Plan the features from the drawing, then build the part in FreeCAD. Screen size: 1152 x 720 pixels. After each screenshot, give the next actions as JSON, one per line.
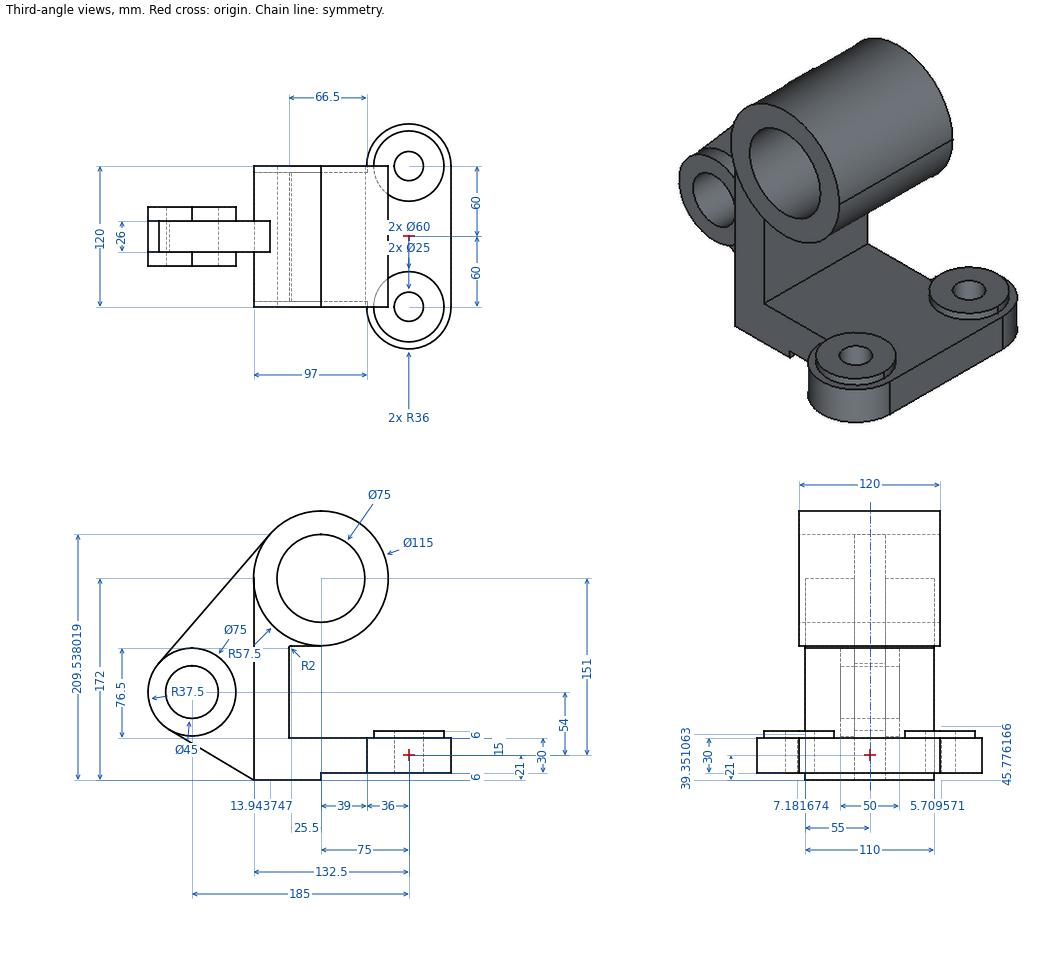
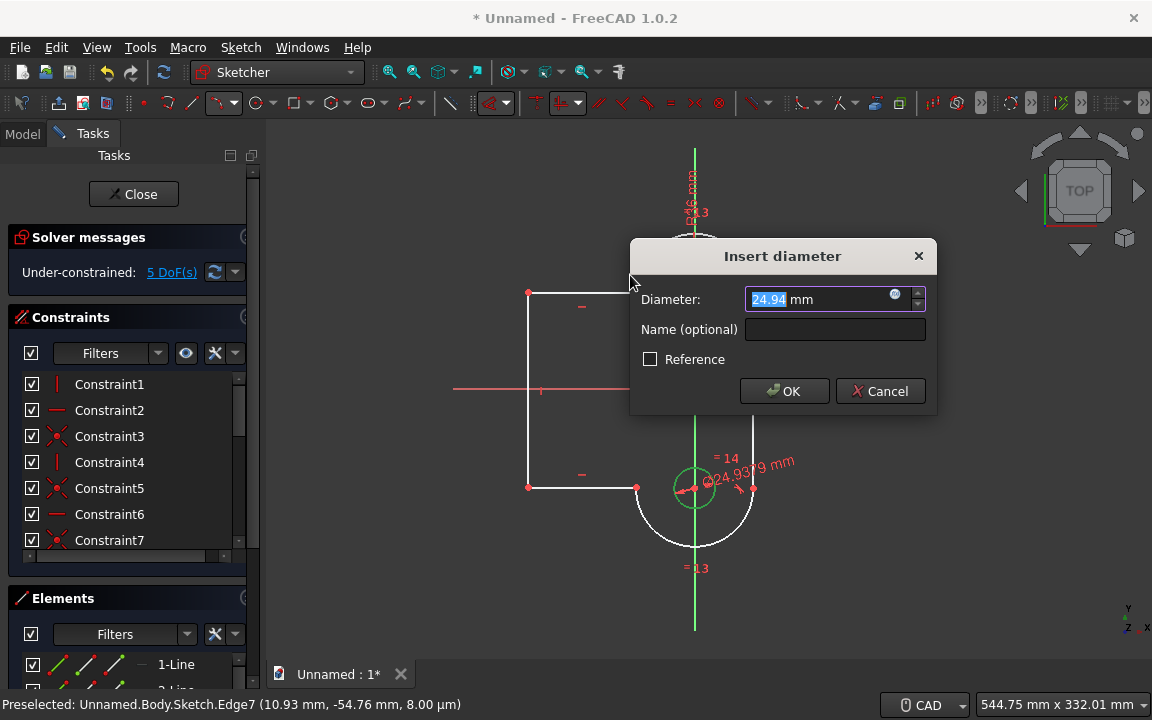
{"action": "type", "text": "25"}
{"action": "key", "text": "Return"}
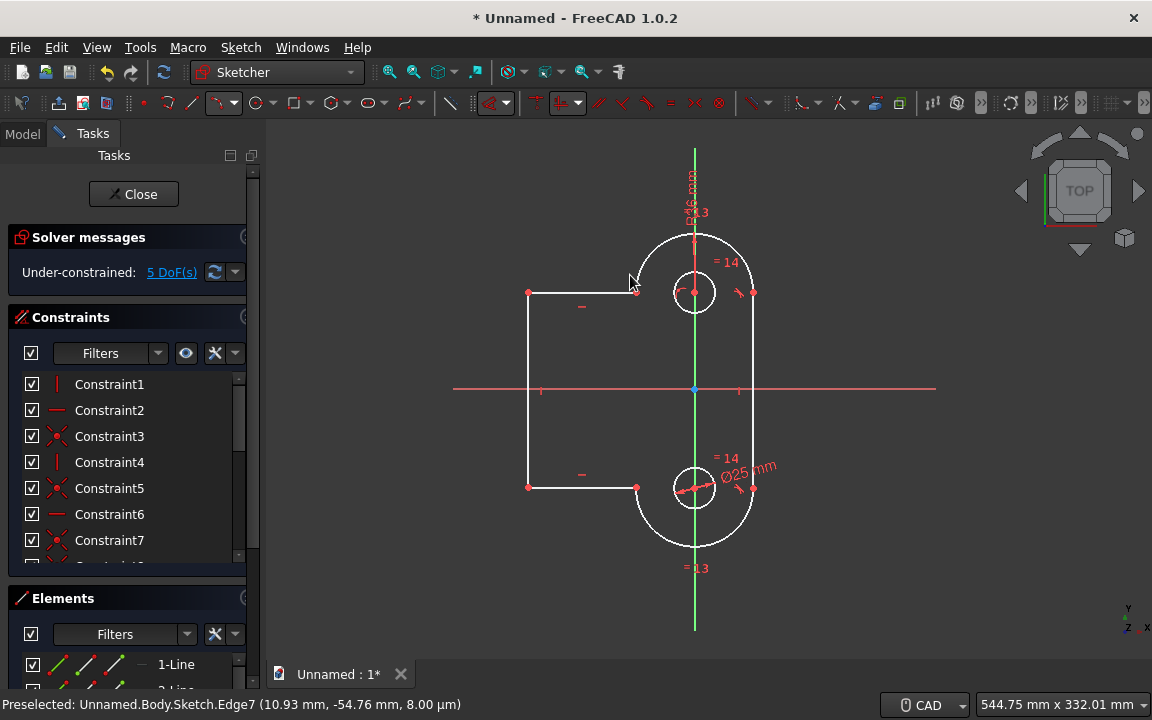
{"action": "left_click", "coordinate": [695, 488]}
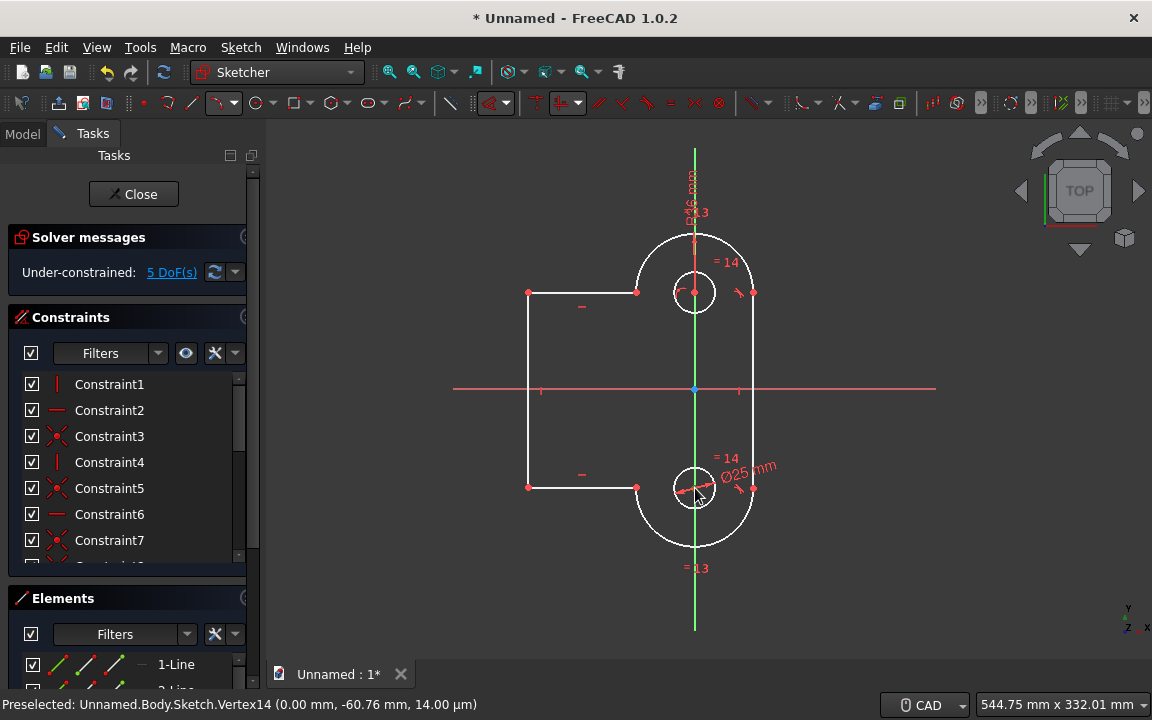
{"action": "key", "text": "i"}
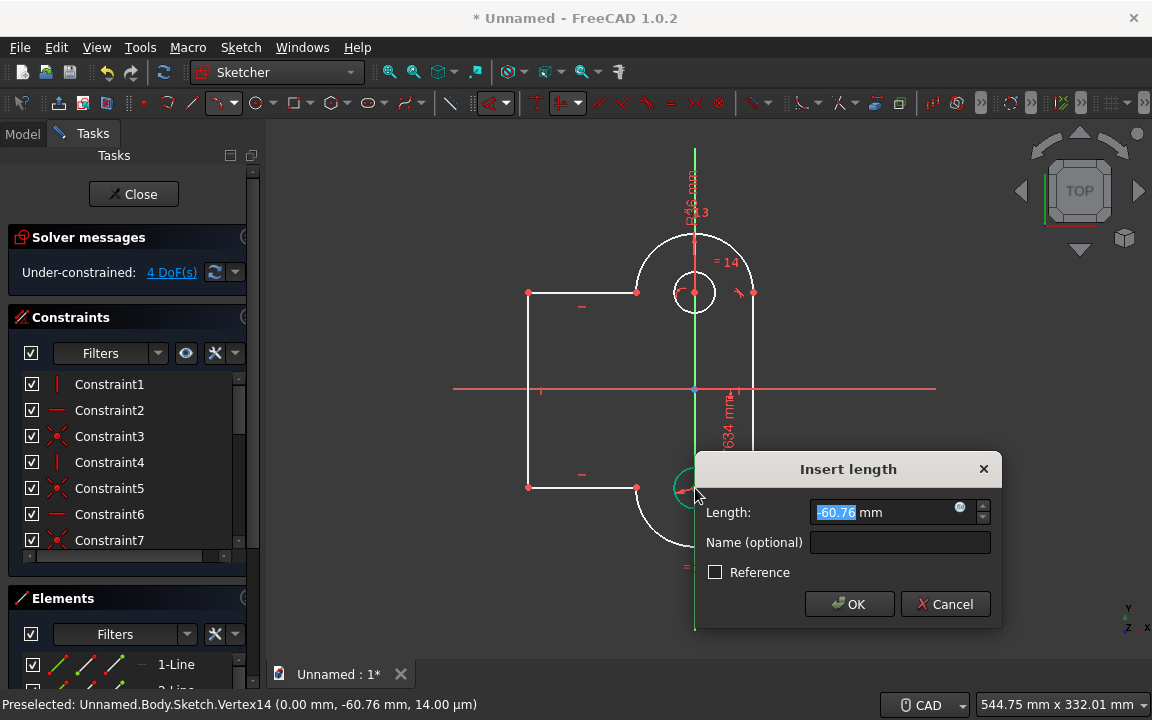
{"action": "type", "text": "-60"}
{"action": "key", "text": "Return"}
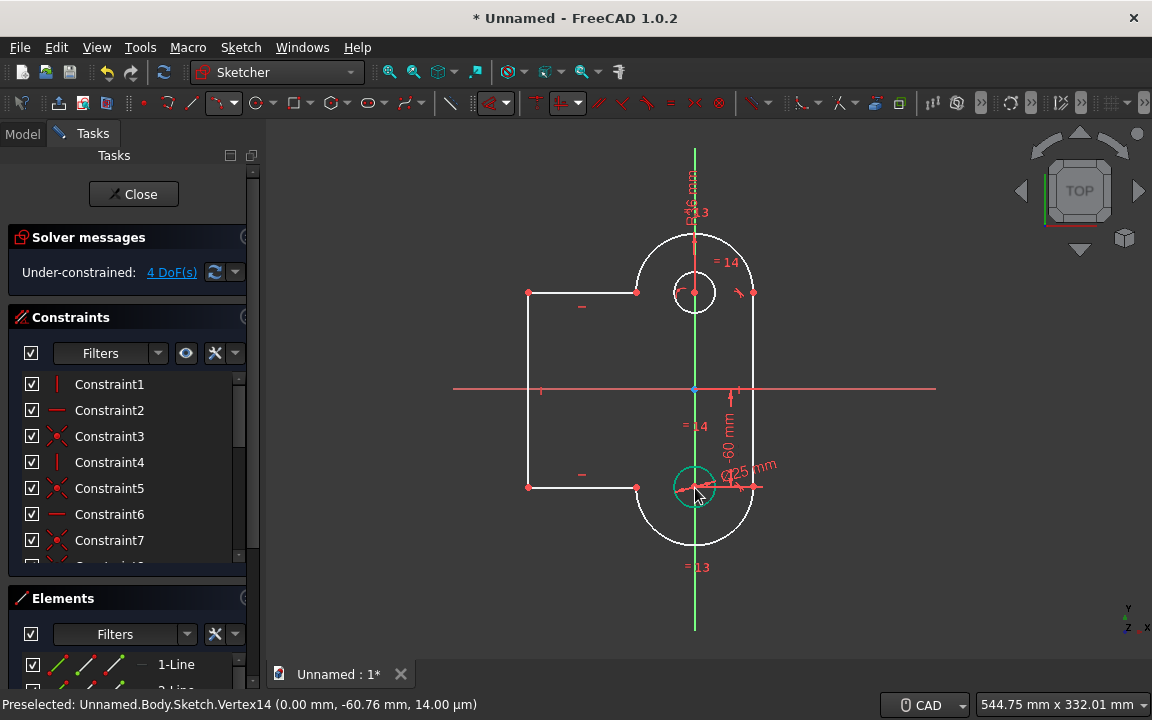
{"action": "left_click", "coordinate": [695, 293]}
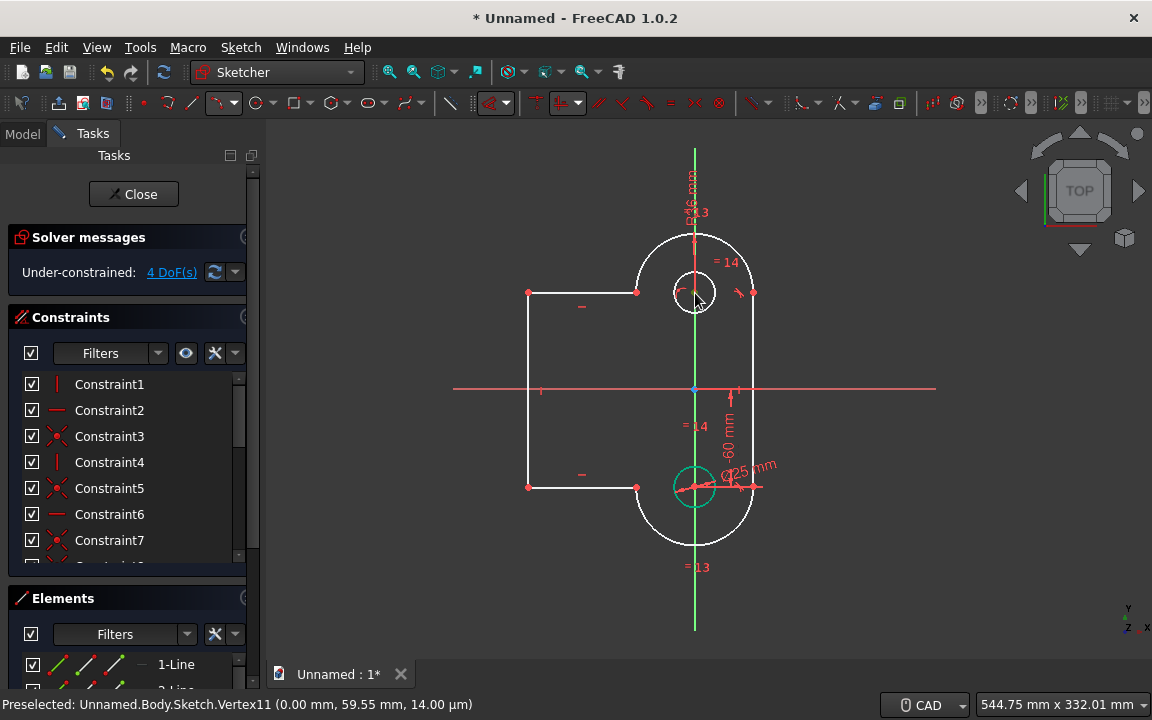
{"action": "key", "text": "i"}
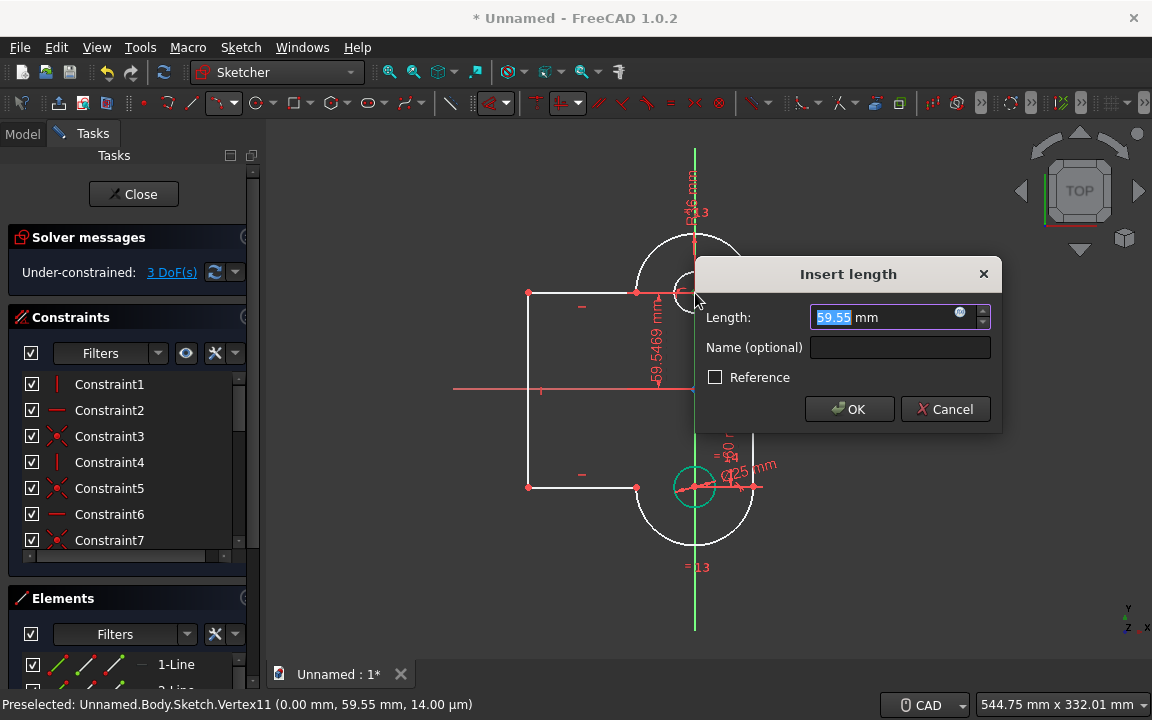
{"action": "type", "text": "60"}
{"action": "key", "text": "Return"}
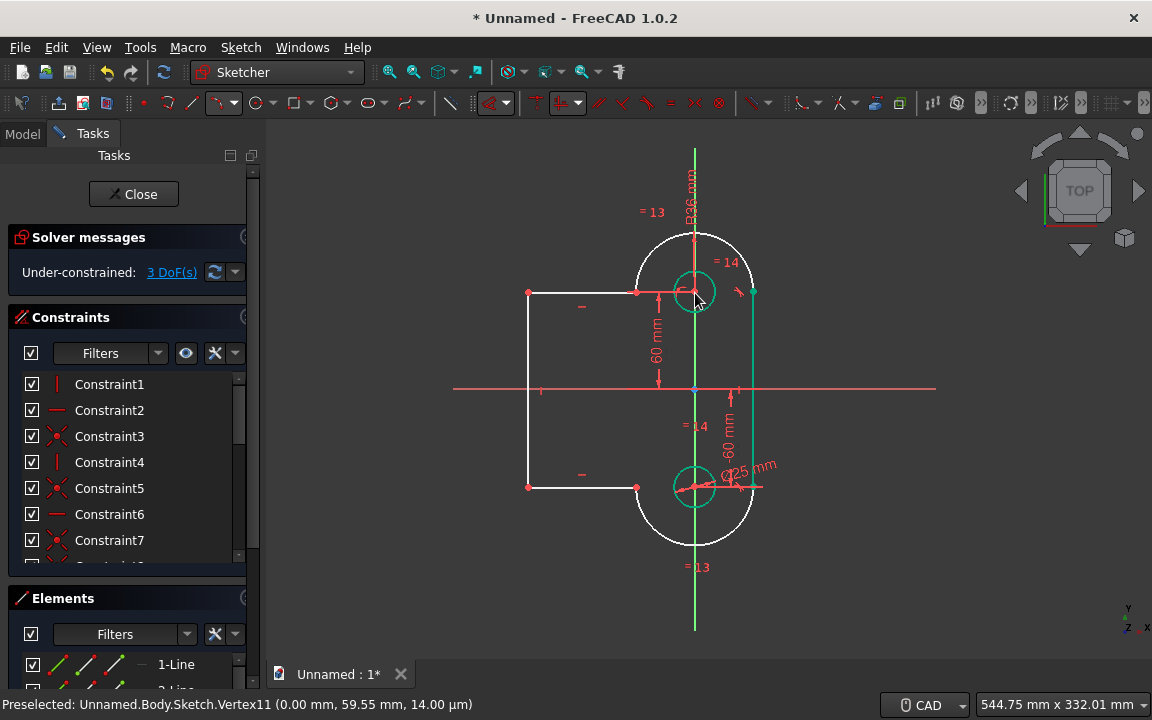
{"action": "left_click", "coordinate": [528, 351]}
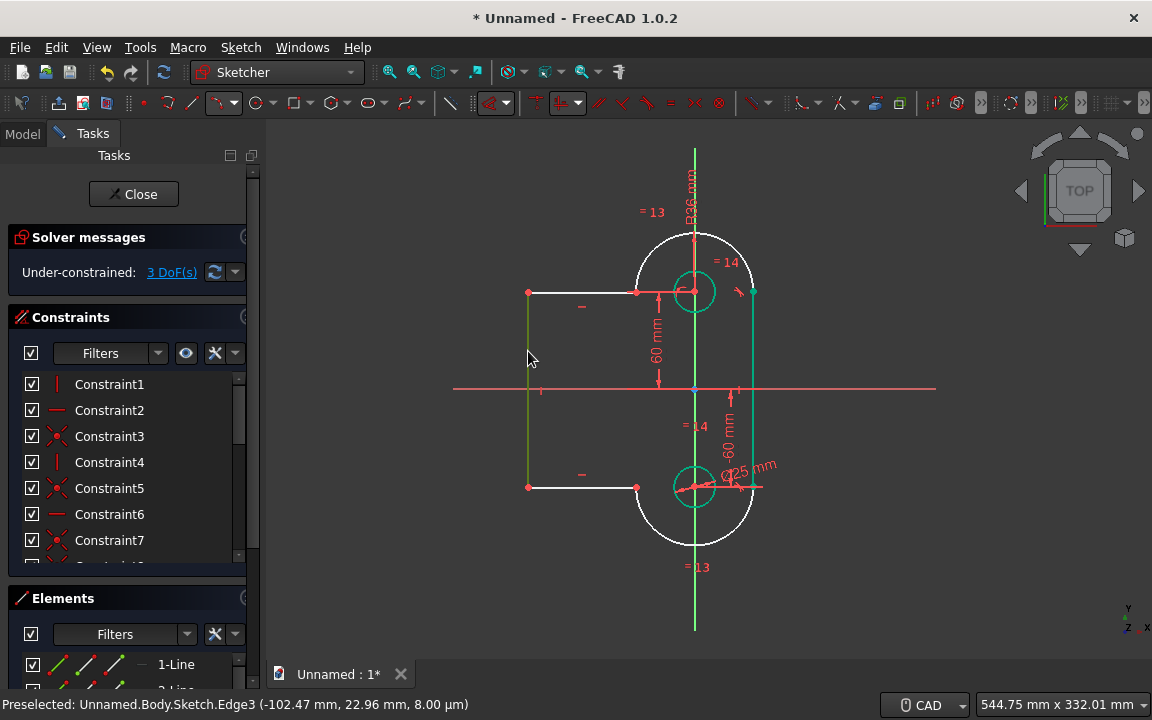
{"action": "key", "text": "i"}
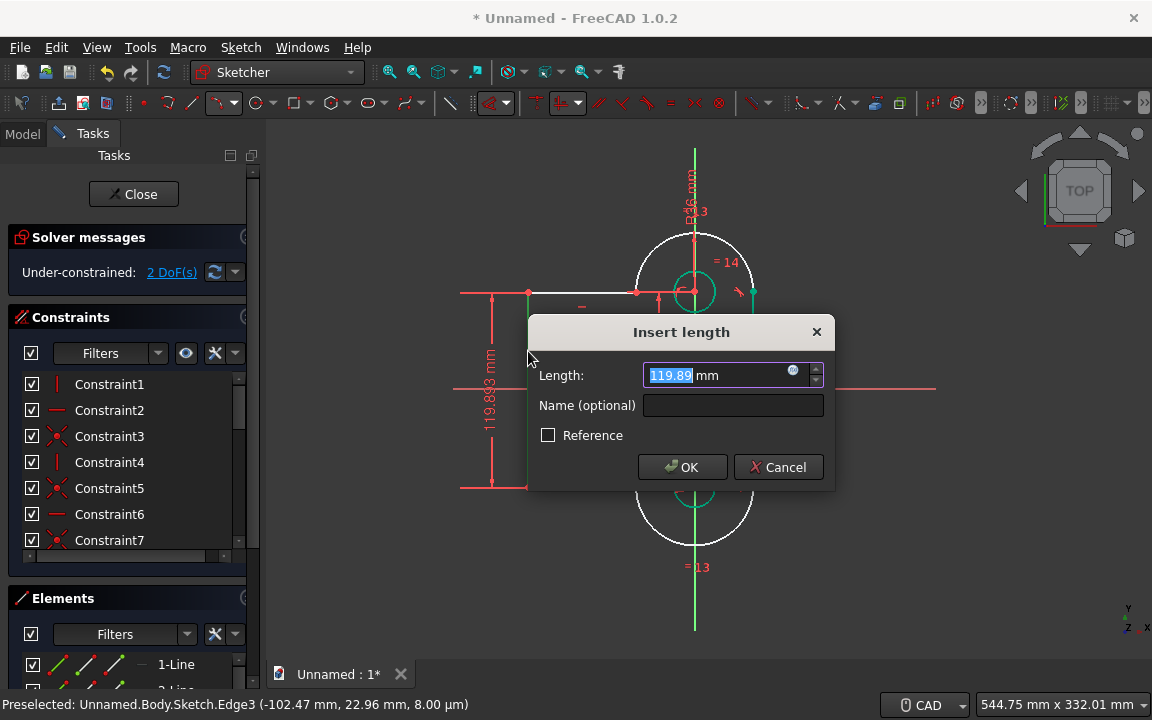
{"action": "type", "text": "120"}
{"action": "key", "text": "Return"}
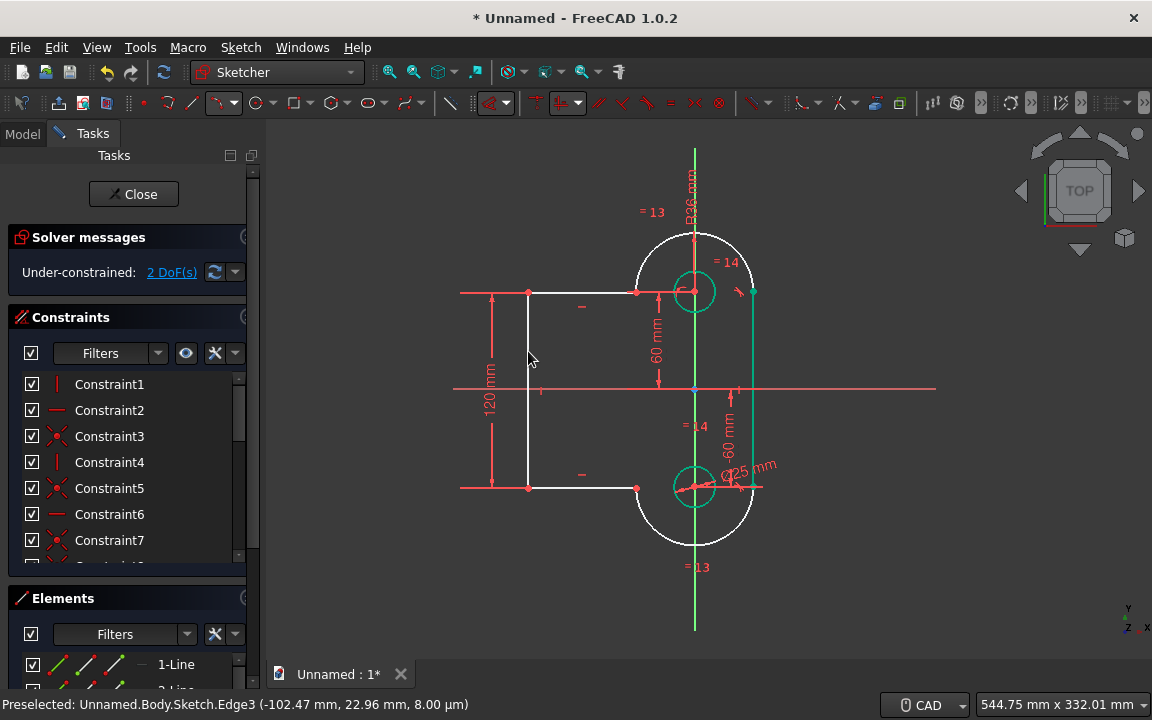
{"action": "left_click", "coordinate": [636, 293]}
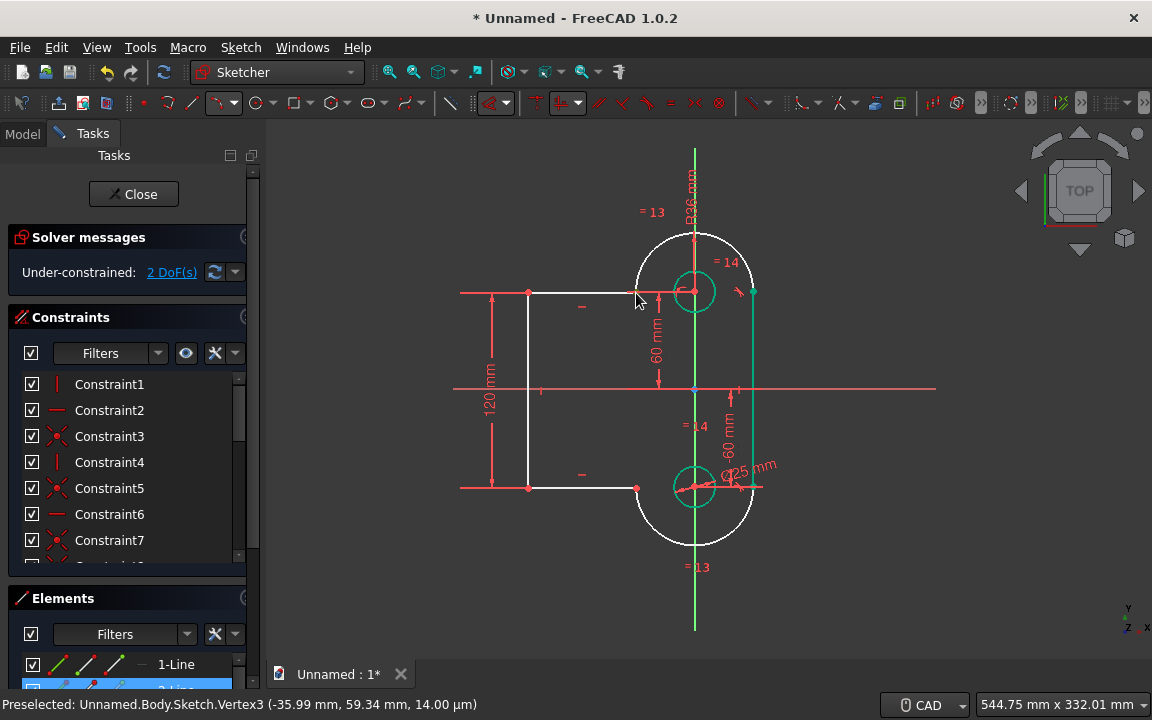
{"action": "key", "text": "i"}